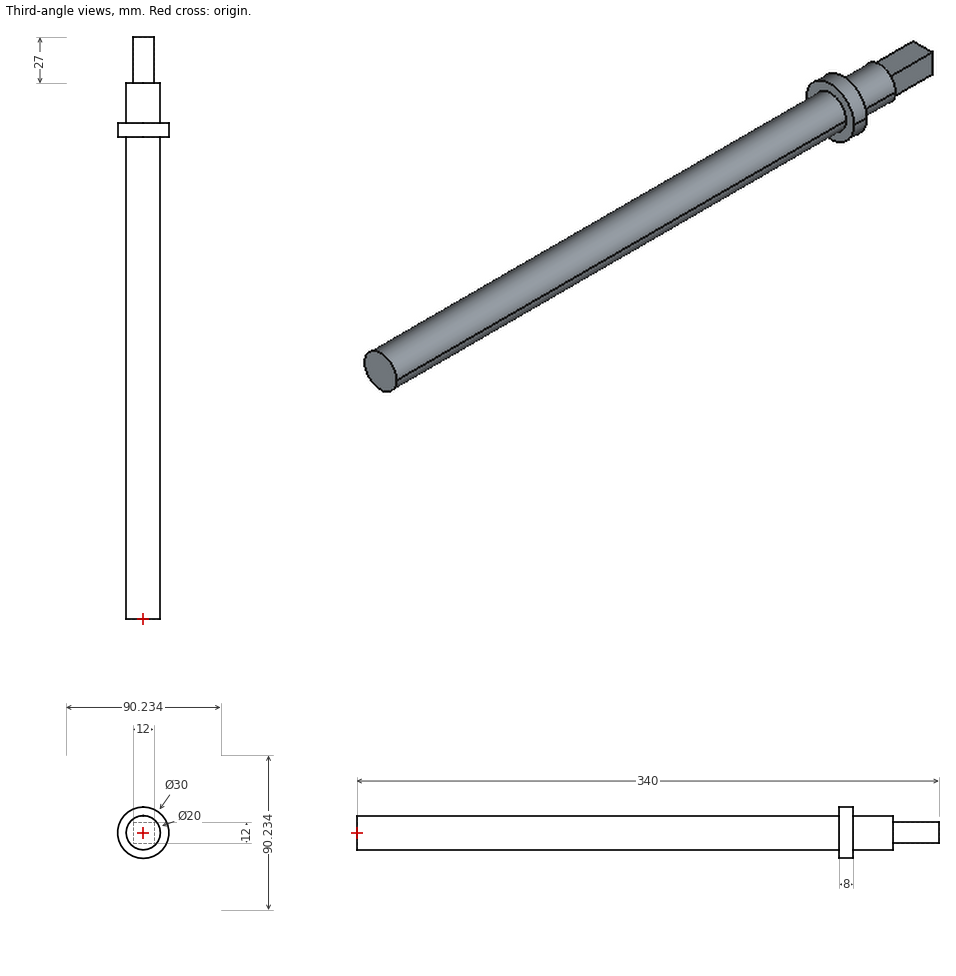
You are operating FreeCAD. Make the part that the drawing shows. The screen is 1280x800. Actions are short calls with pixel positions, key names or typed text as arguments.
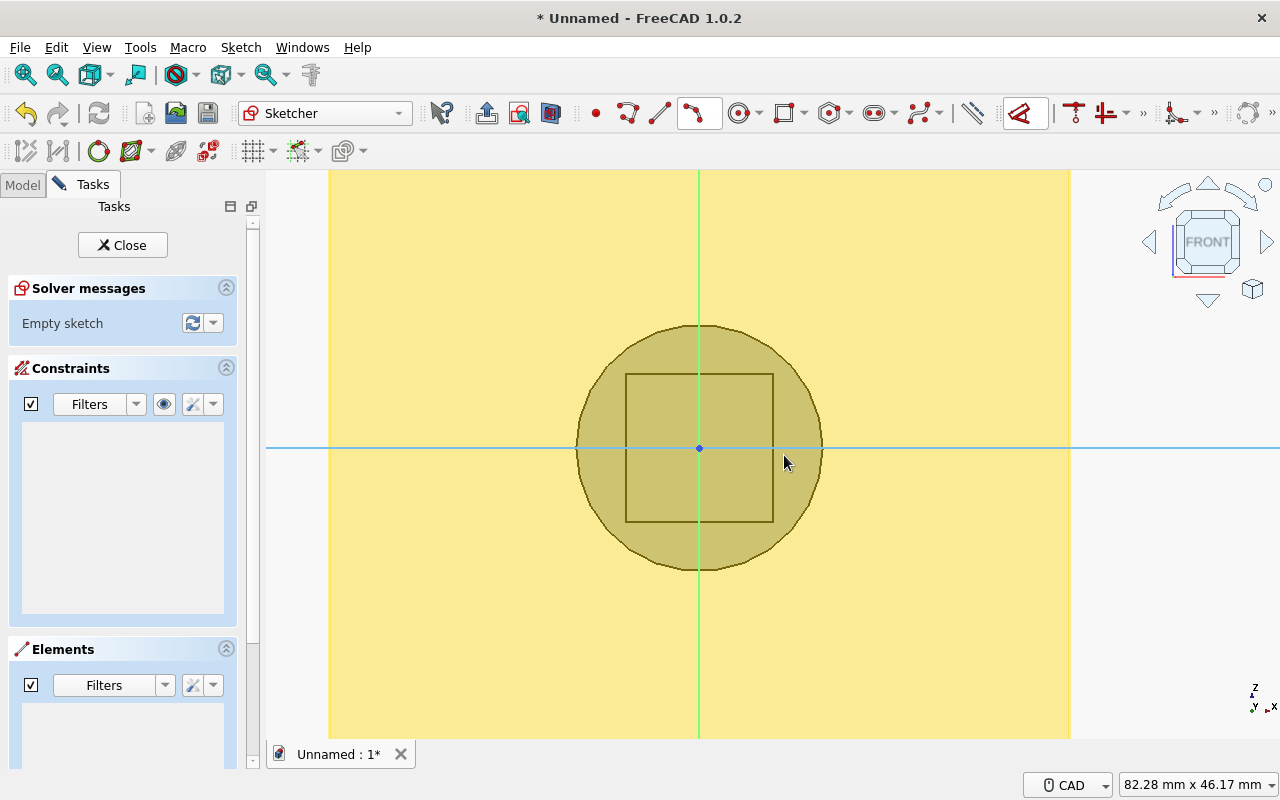
click(740, 114)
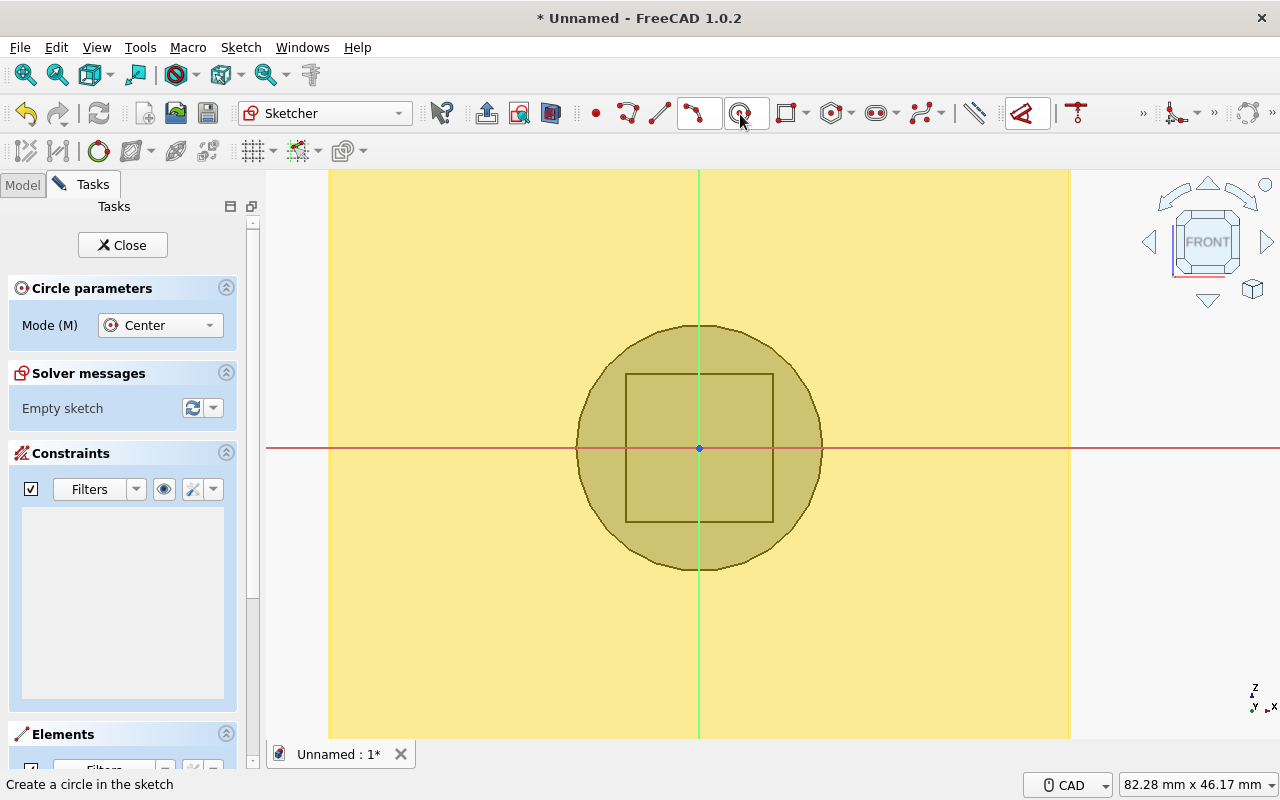
click(699, 448)
move(830, 317)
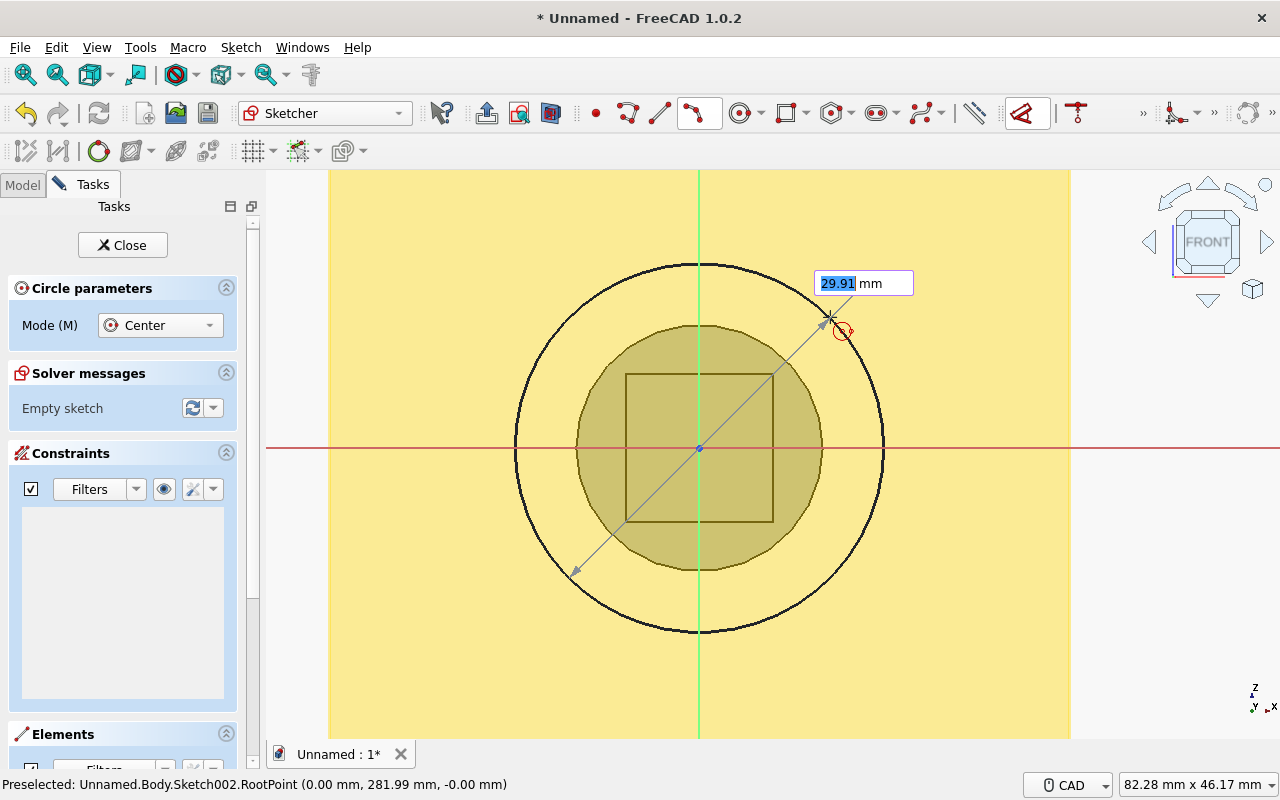
text(30)
key(Return)
key(Escape)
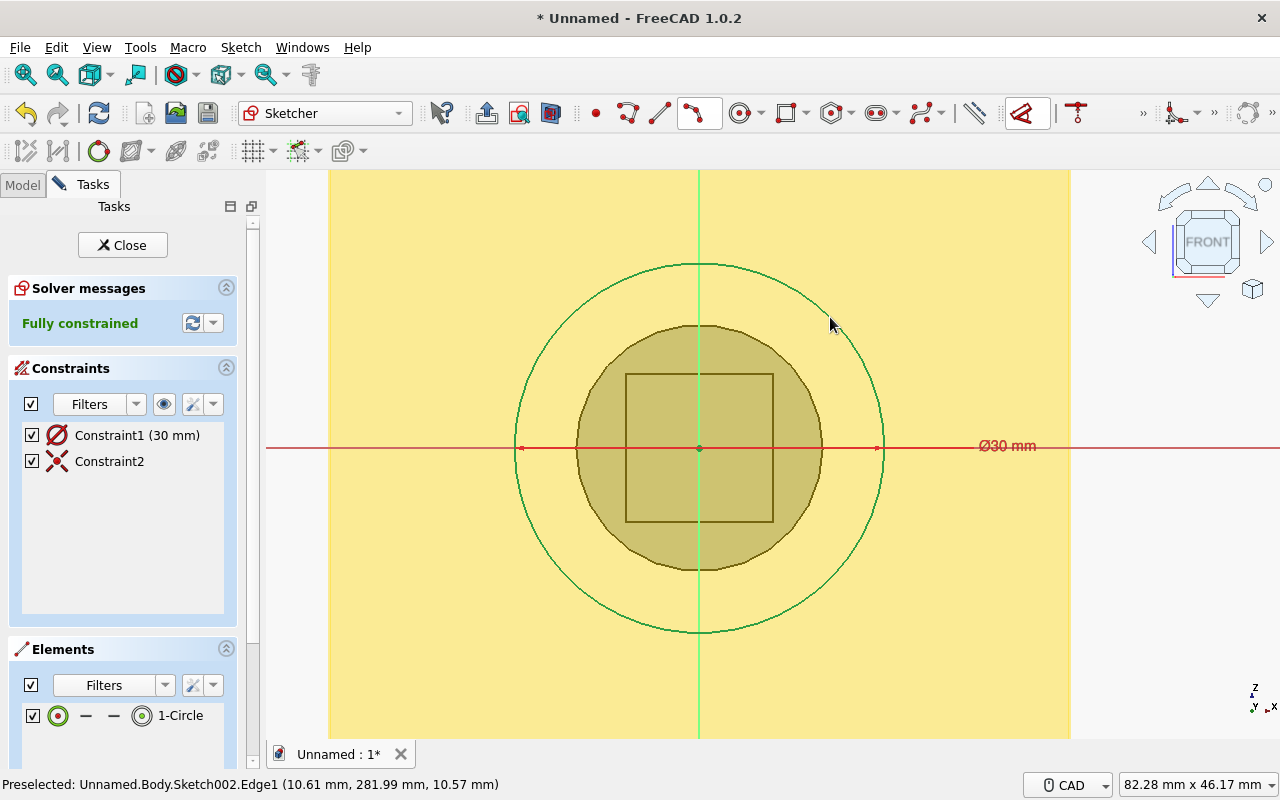
click(123, 245)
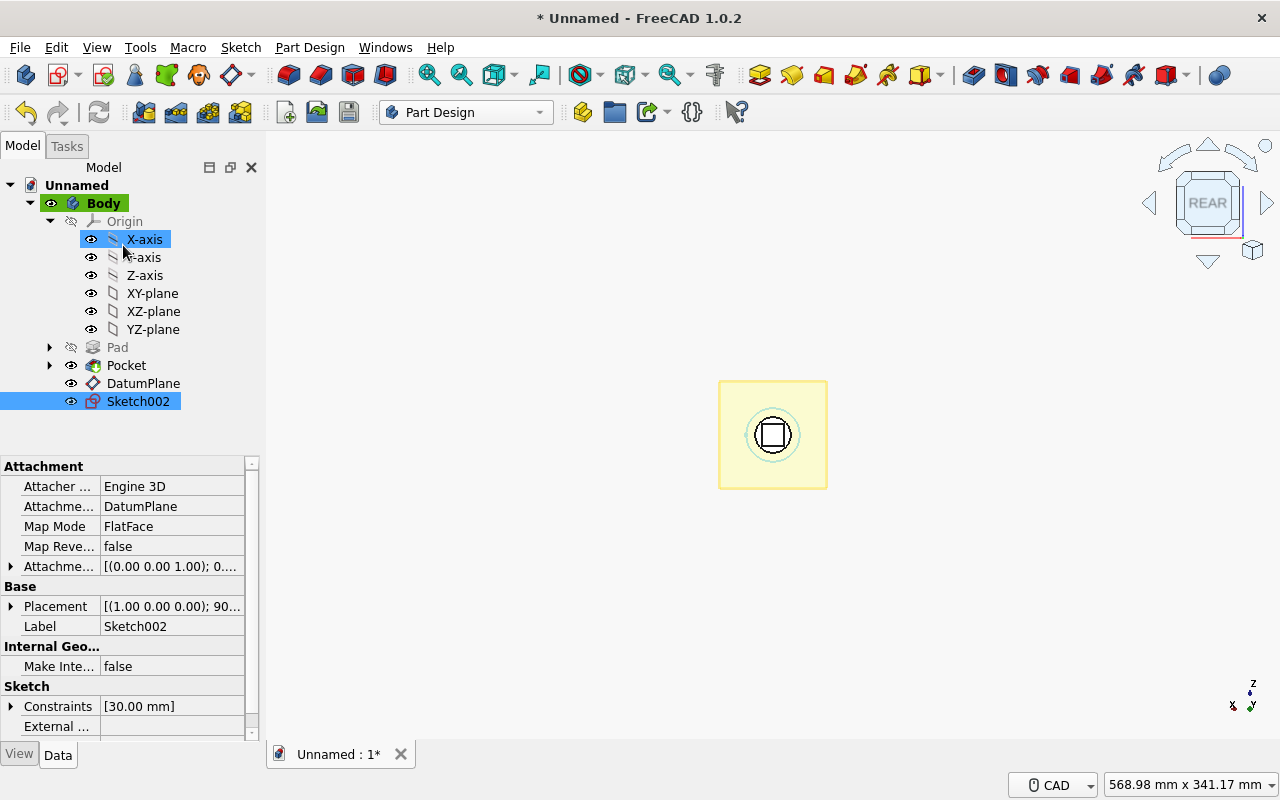
click(760, 76)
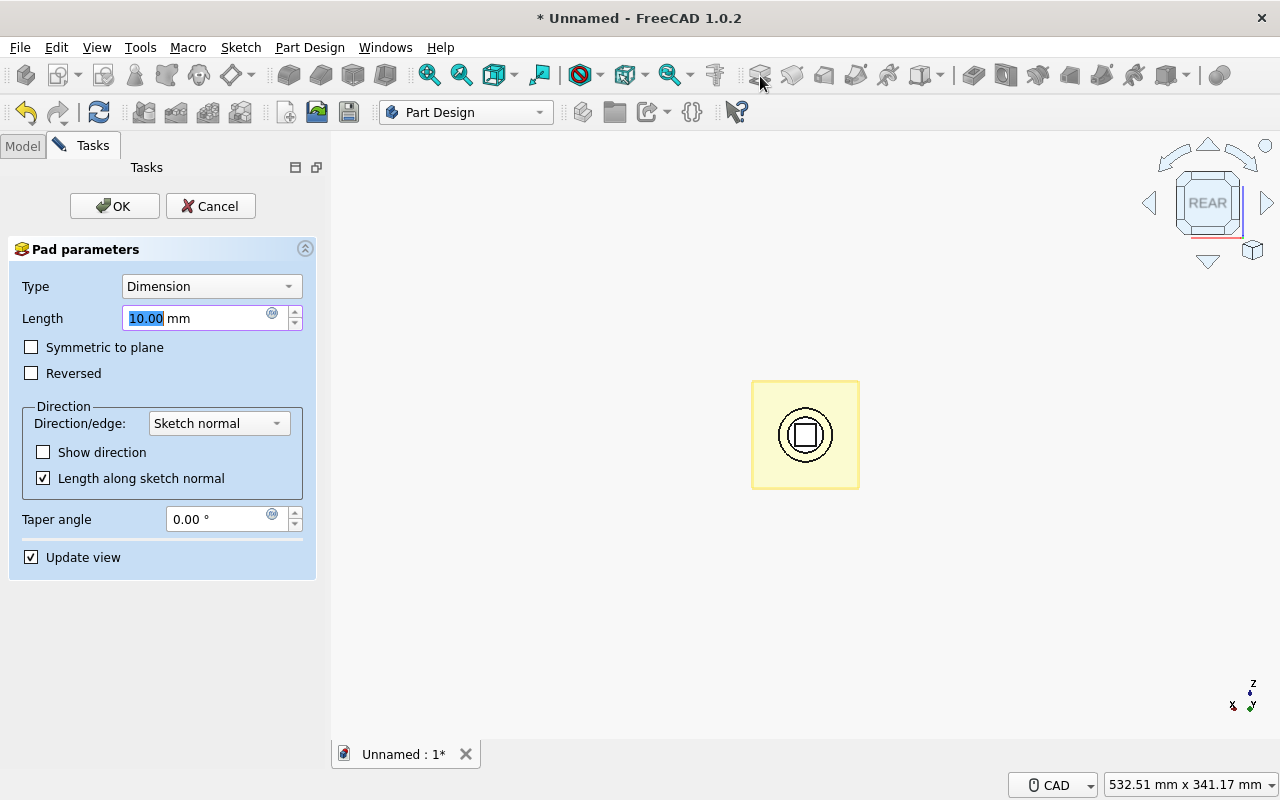
text(8)
key(Tab)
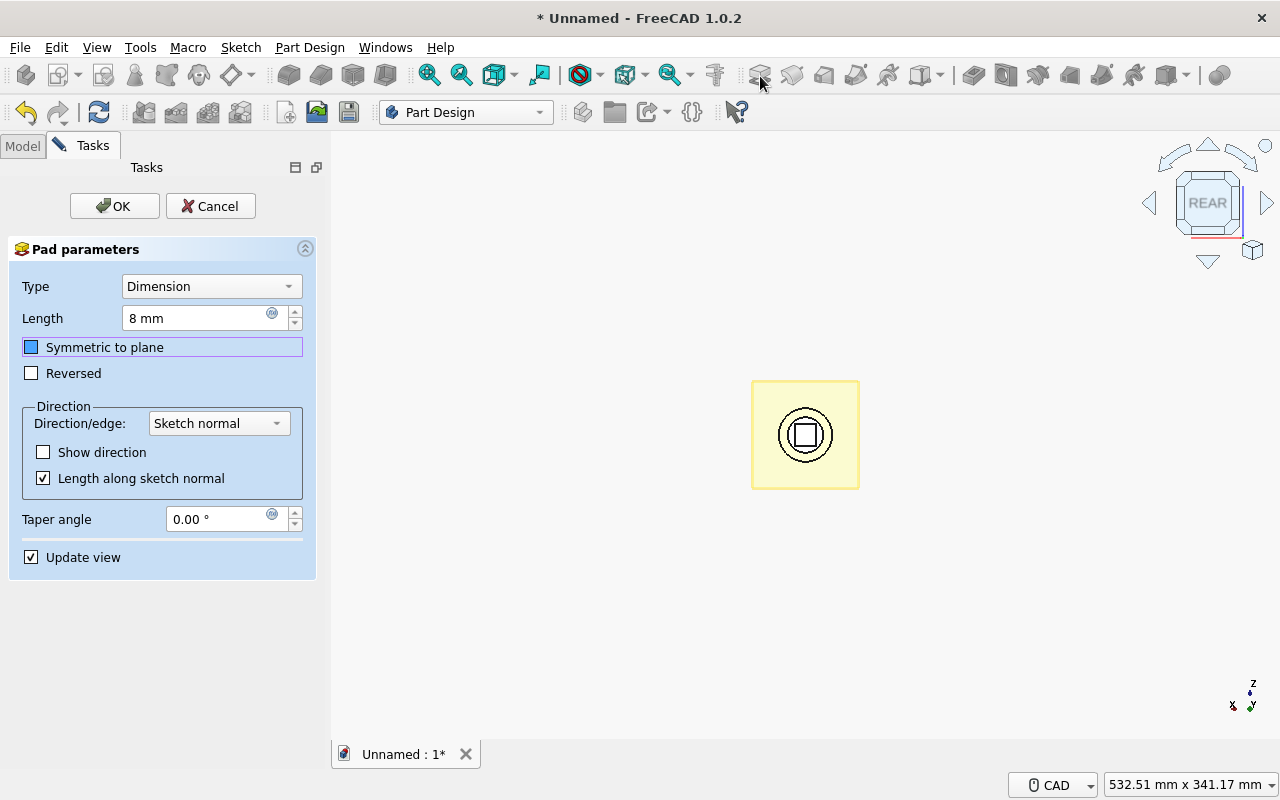
click(30, 373)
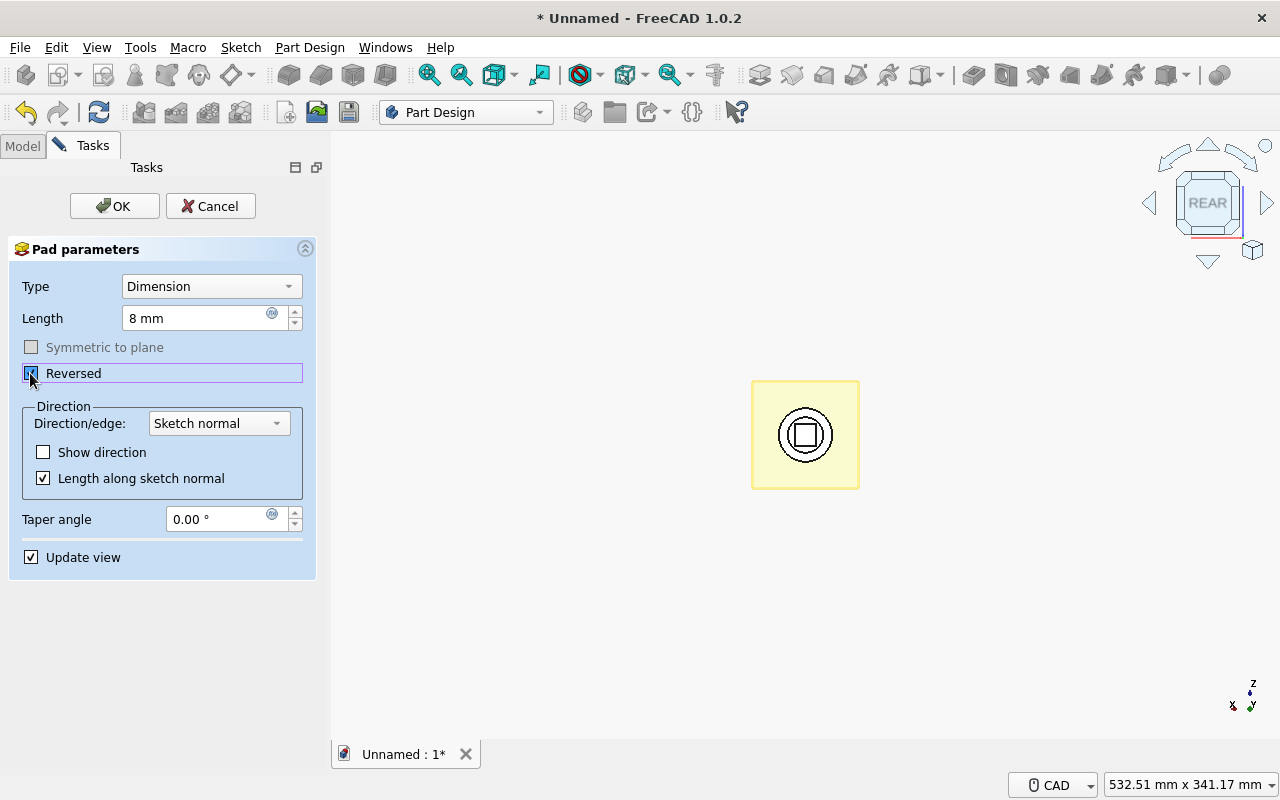
click(115, 206)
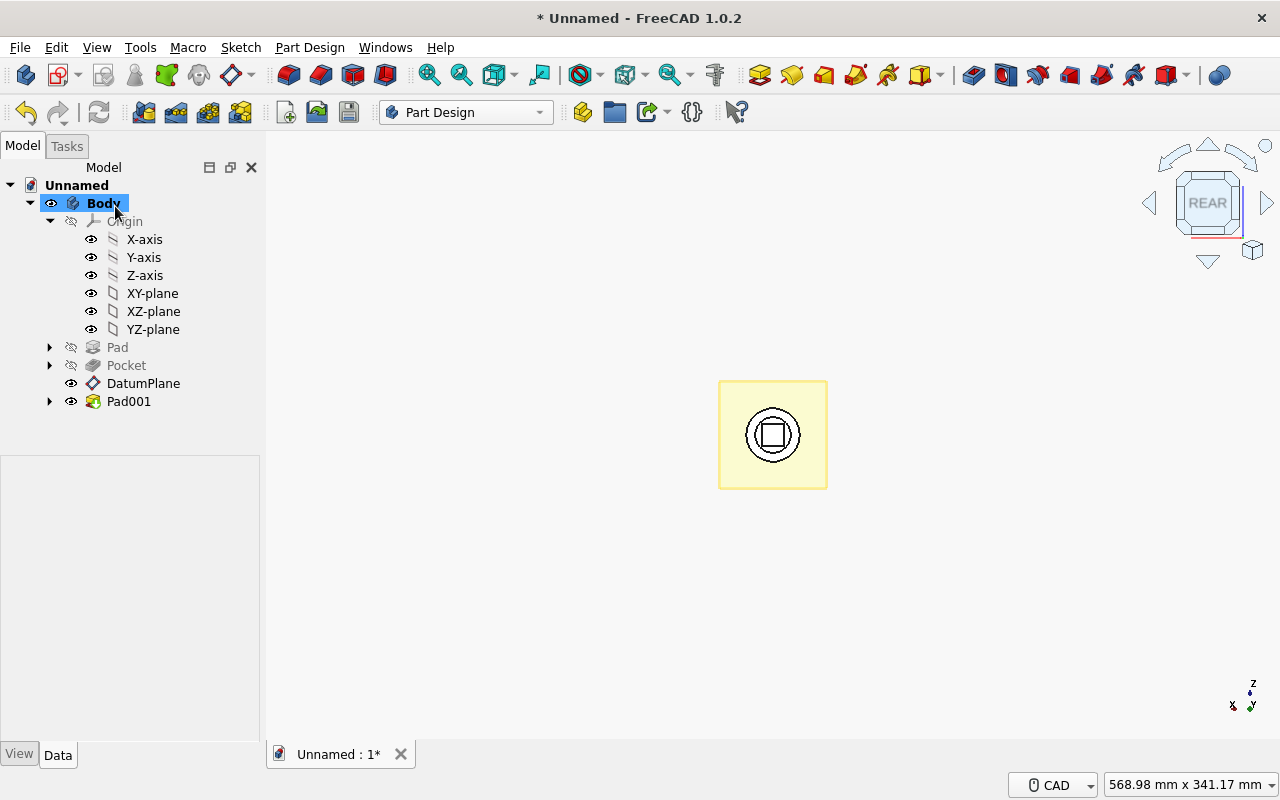
click(116, 383)
key(space)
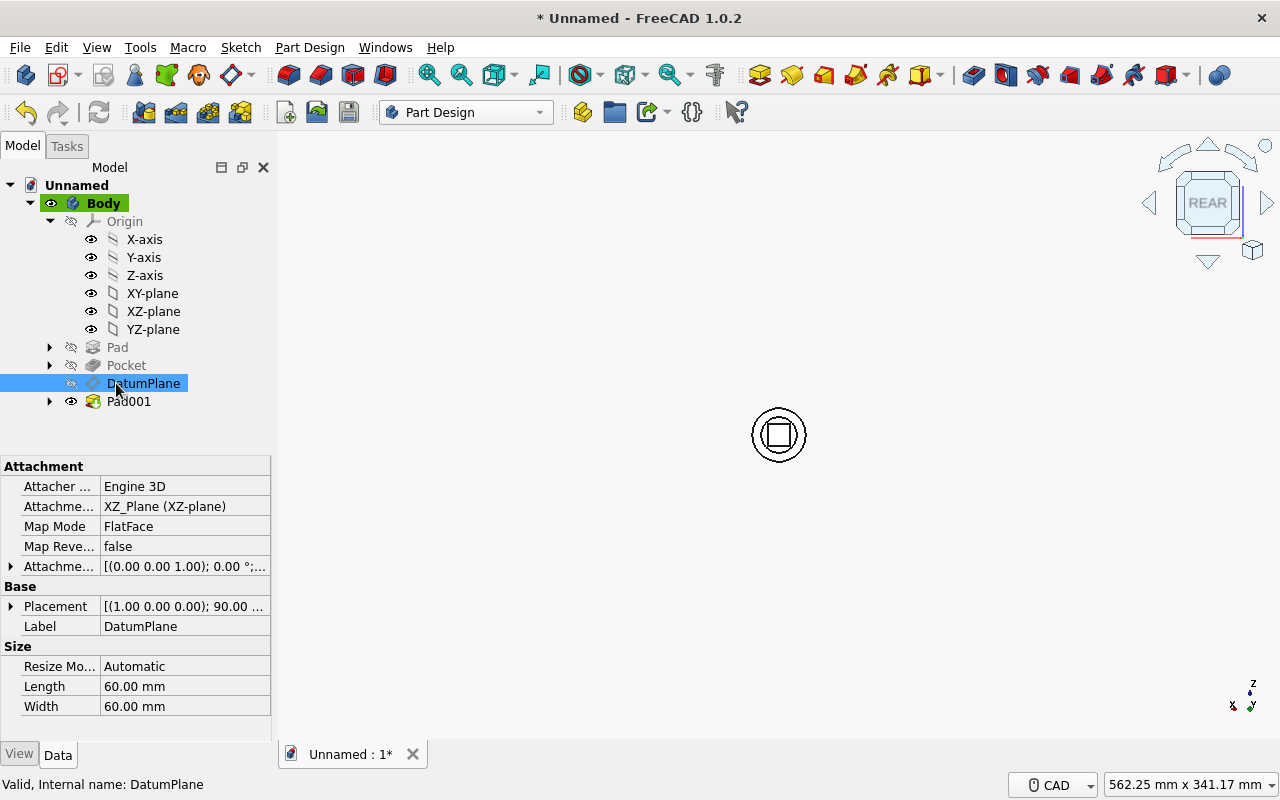
key(0)